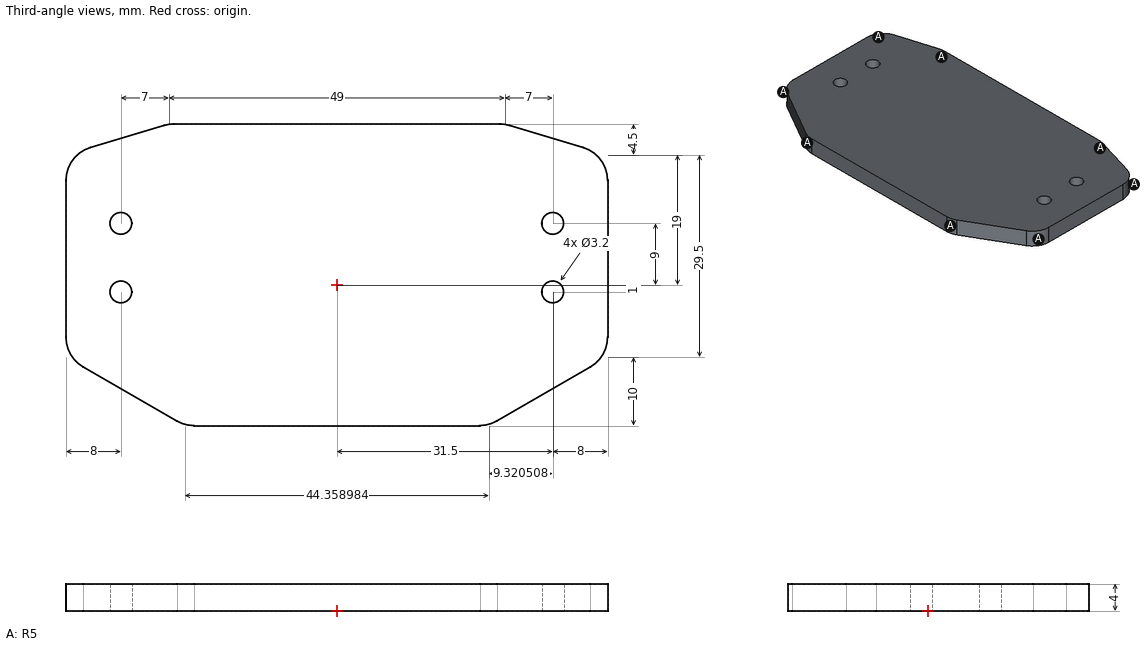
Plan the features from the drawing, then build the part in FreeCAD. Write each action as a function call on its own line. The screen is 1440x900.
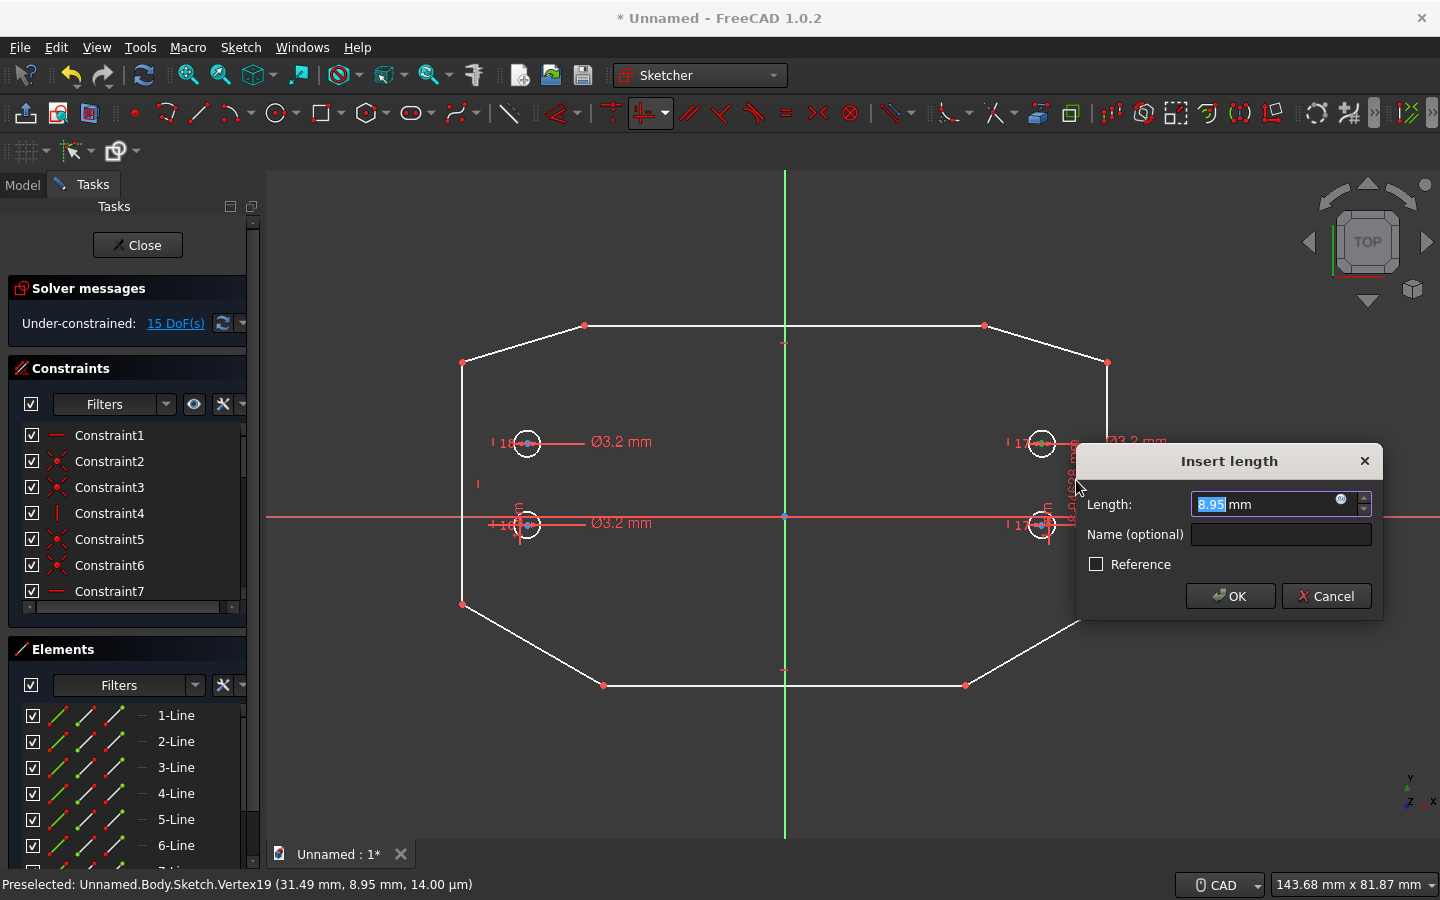
text(9)
key(Return)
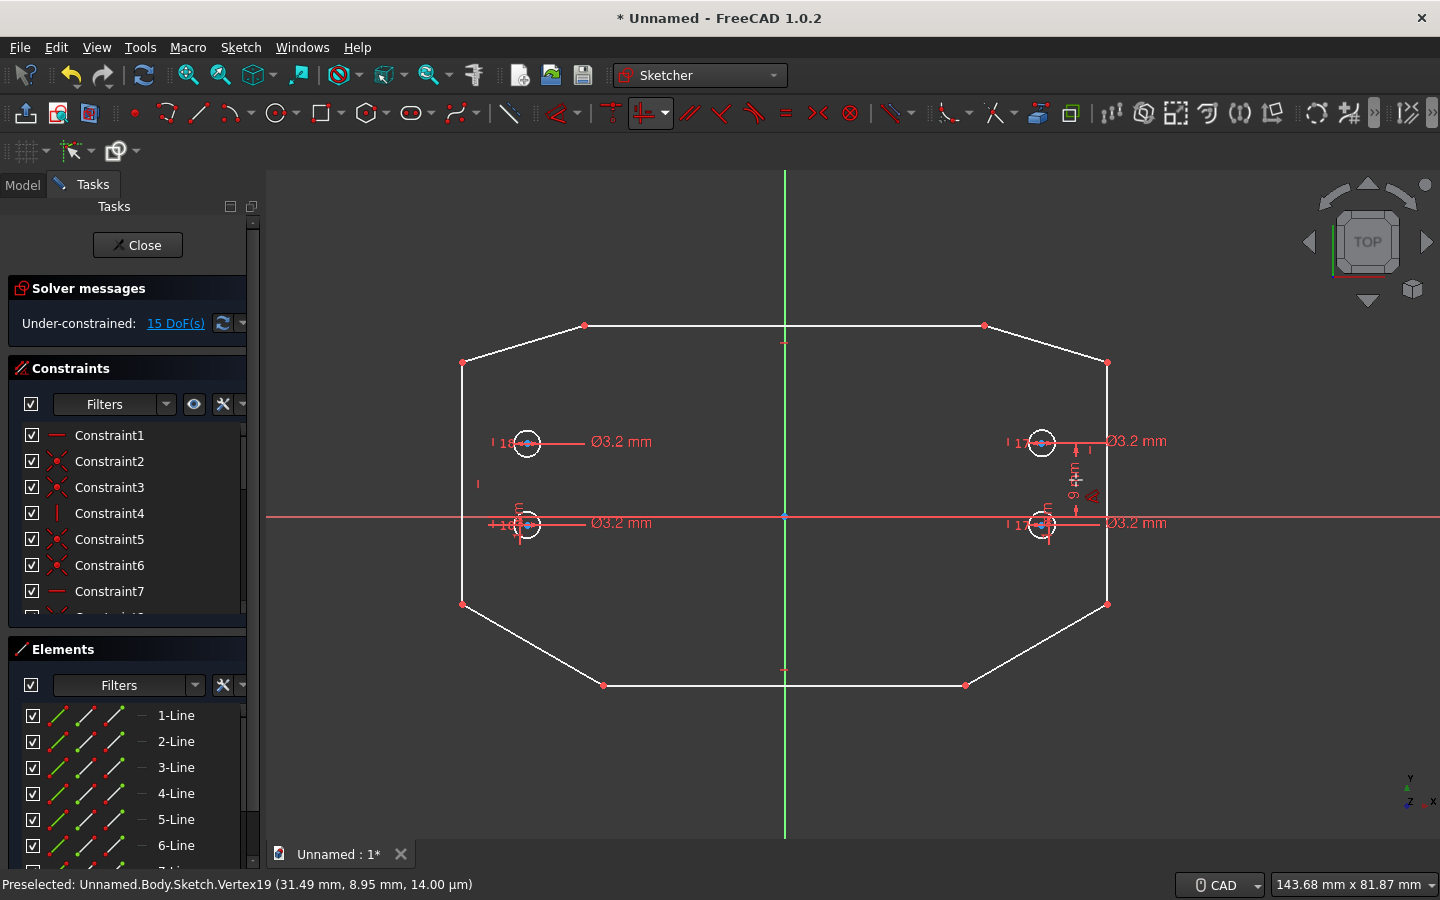
click(527, 444)
click(493, 480)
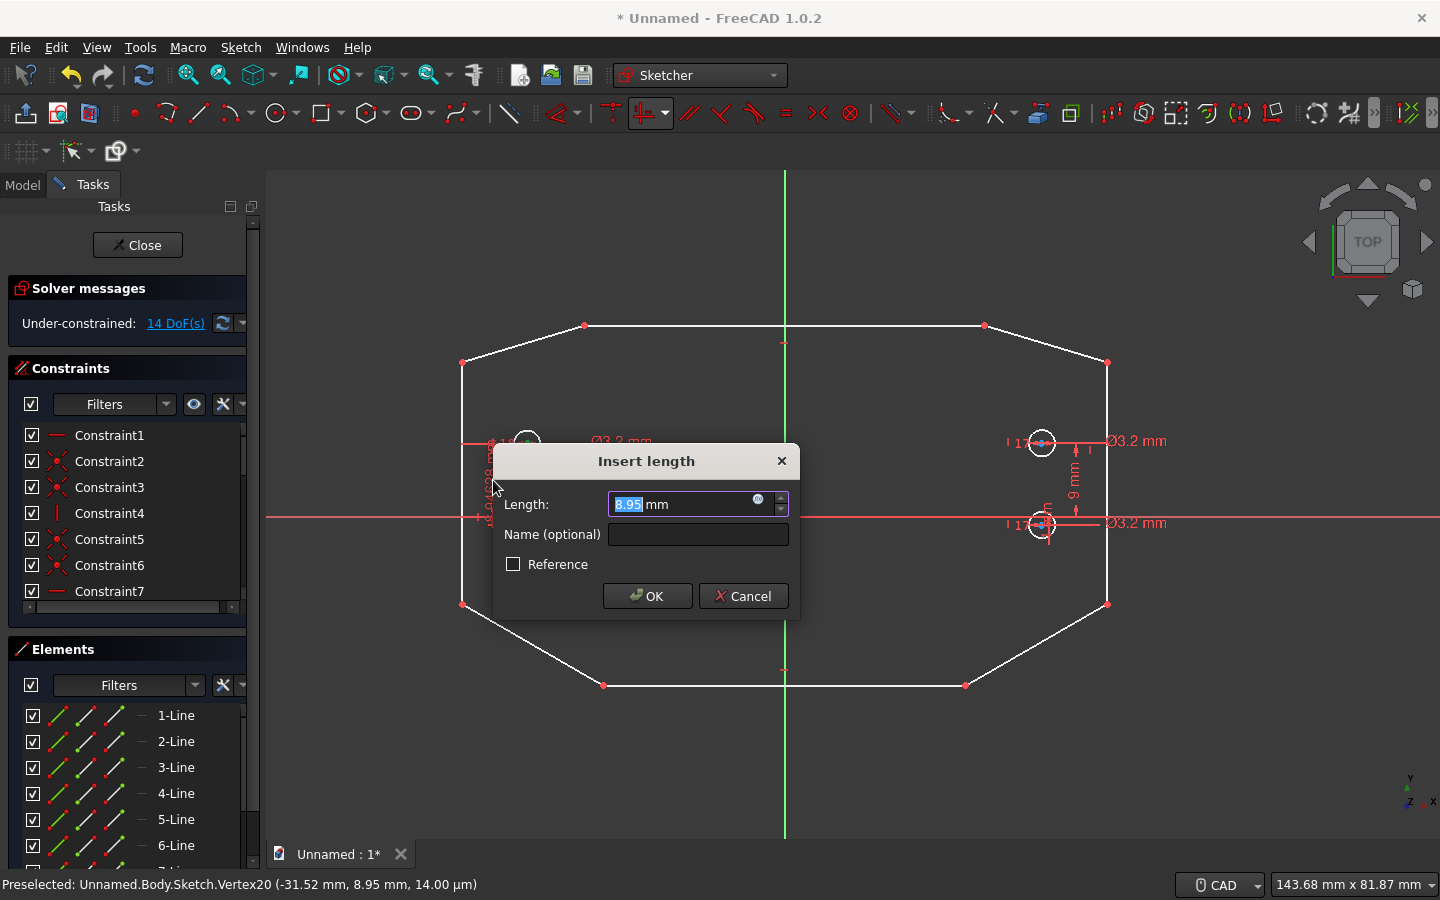
text(9)
key(Return)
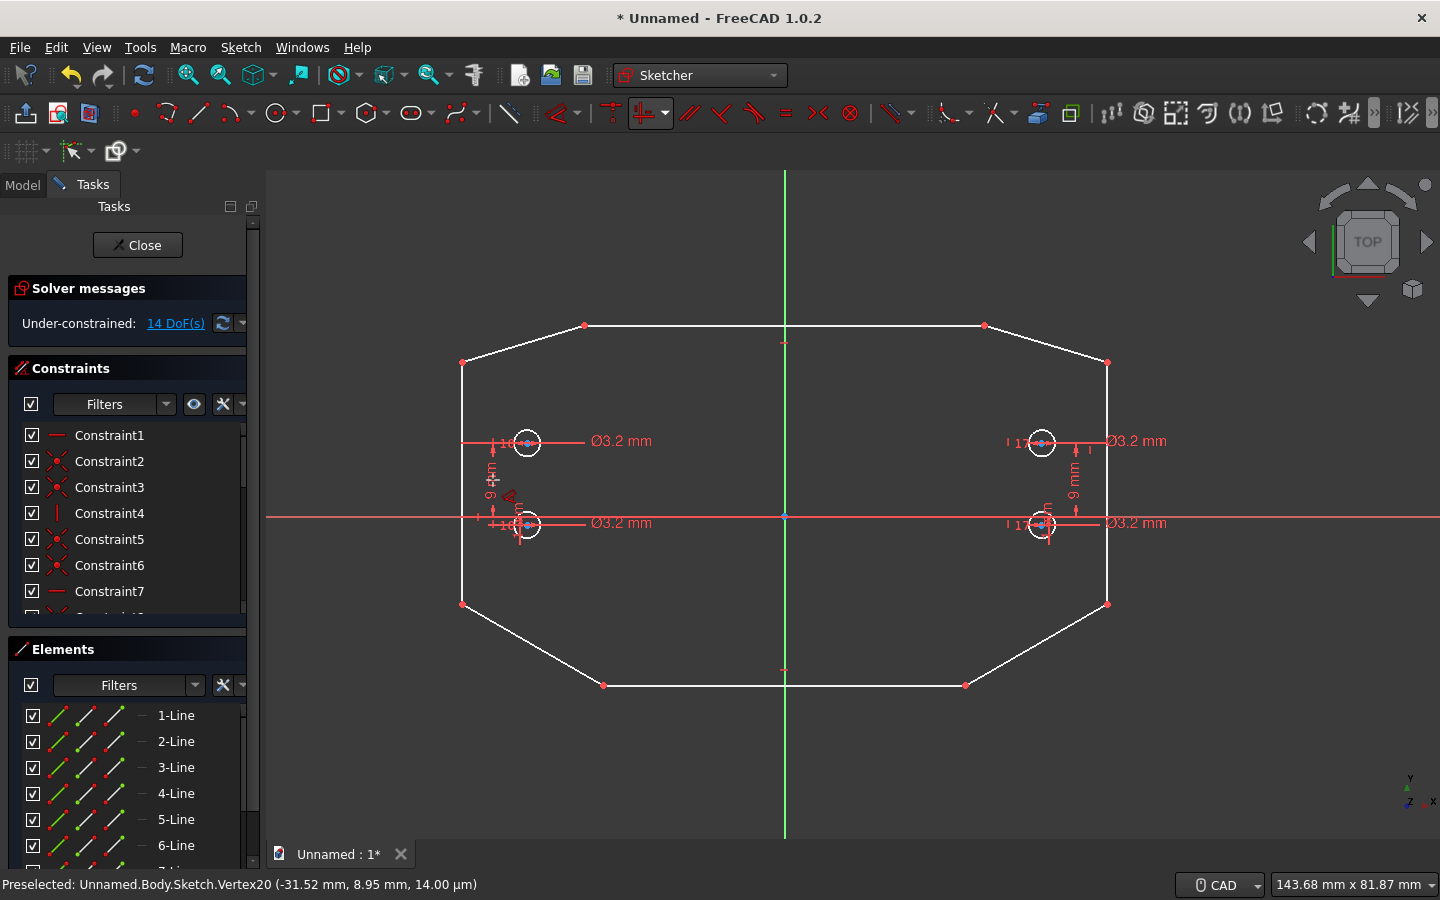
click(865, 326)
click(692, 292)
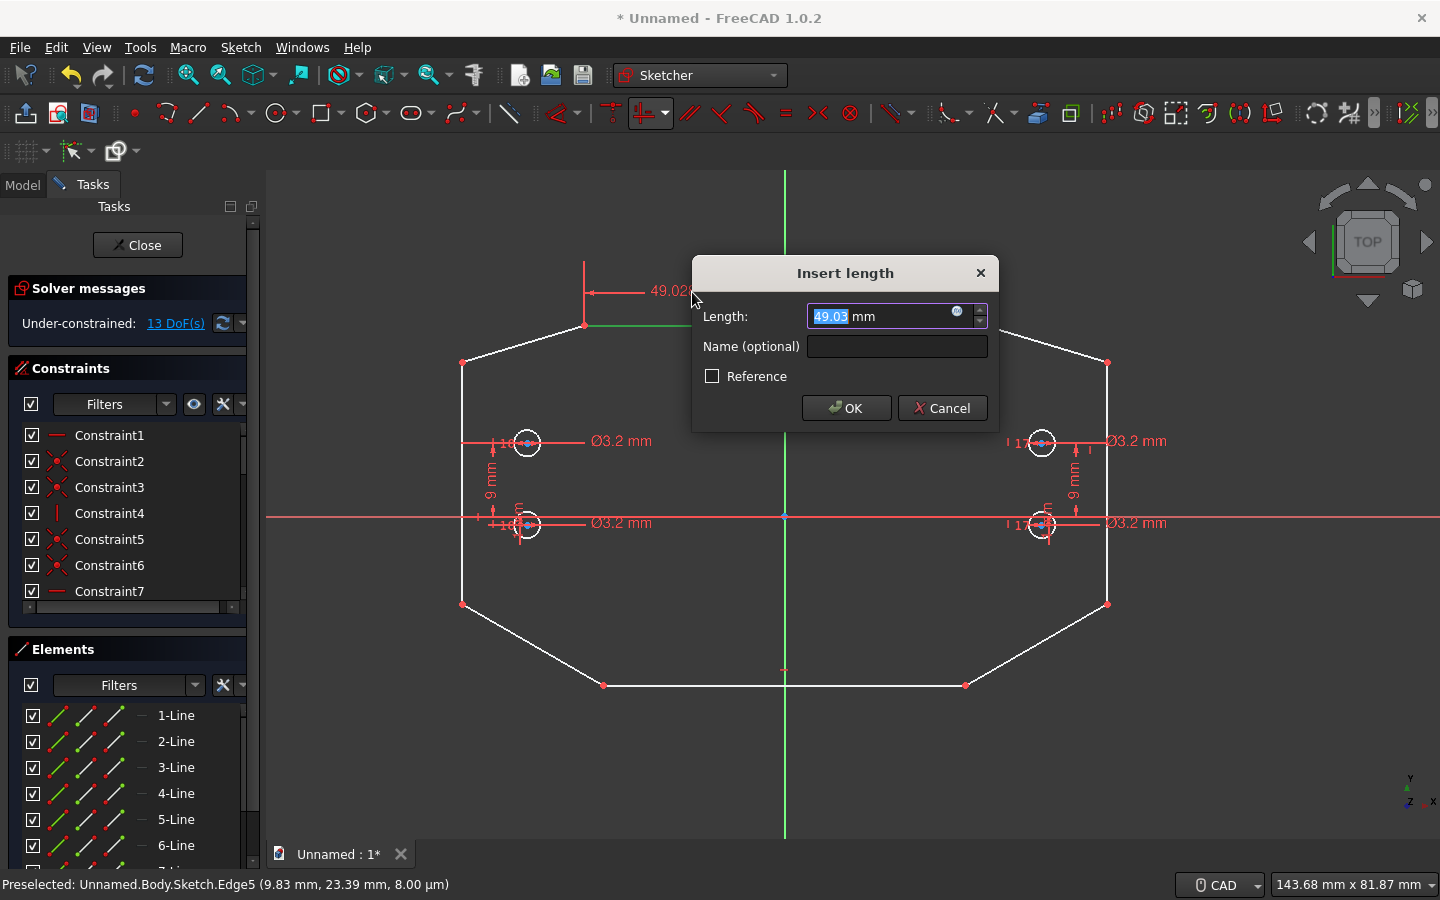
text(49)
key(Return)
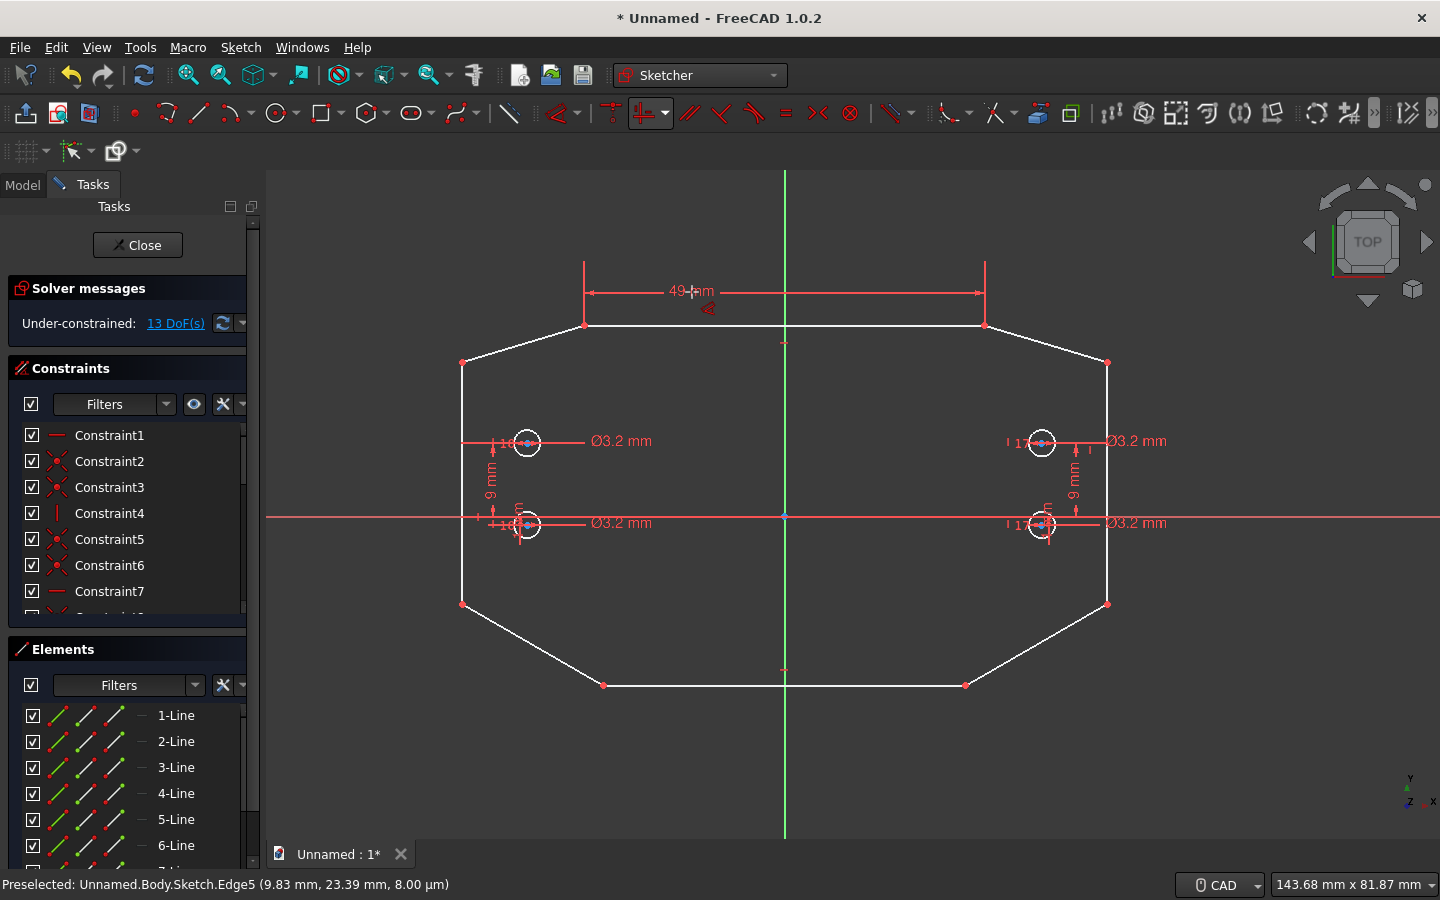
click(1107, 604)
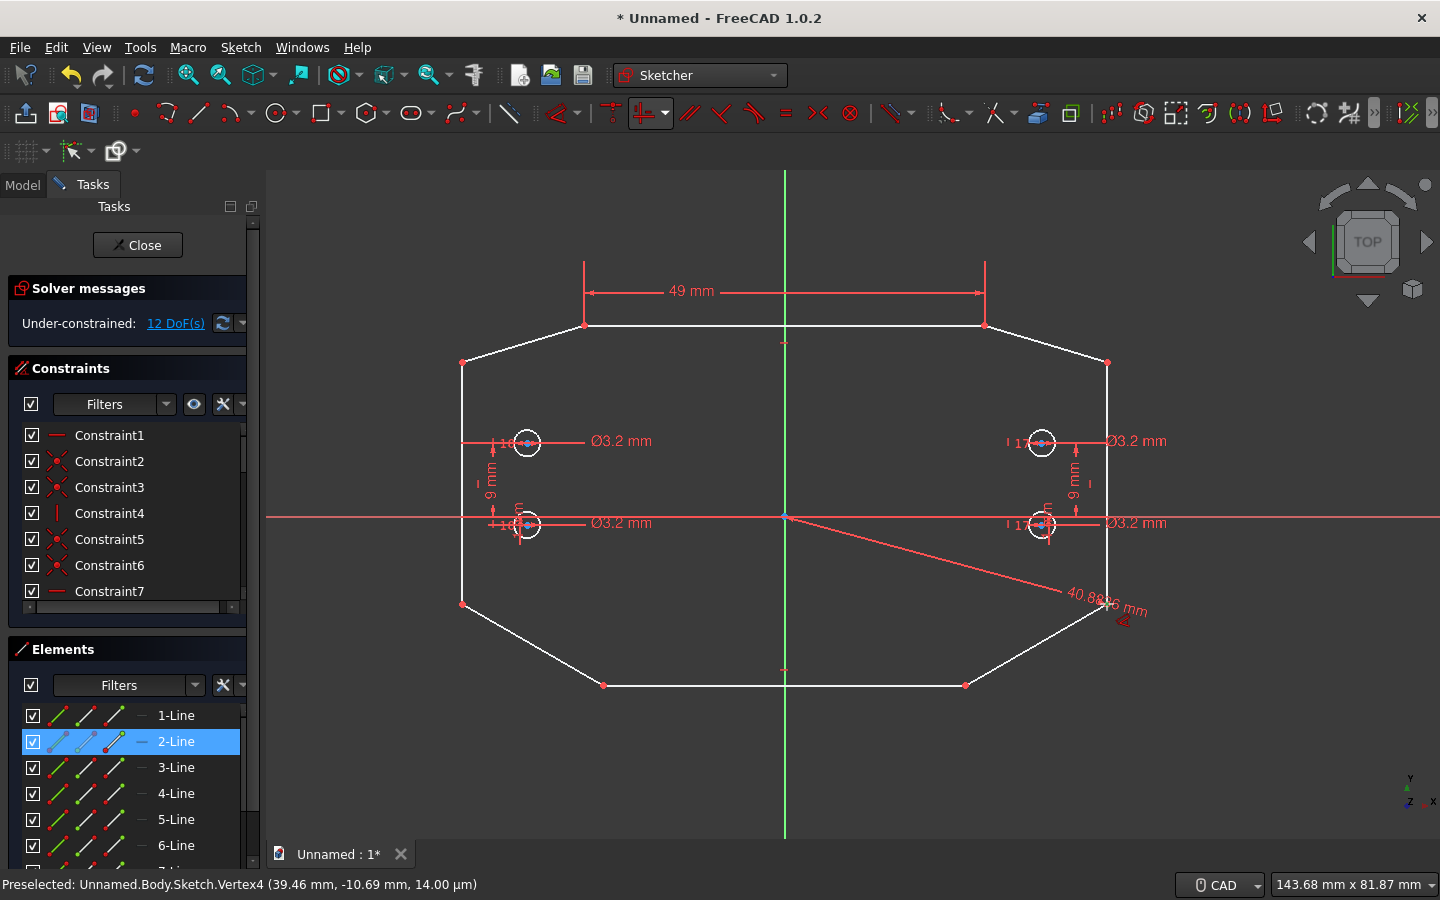
click(1042, 525)
click(1075, 638)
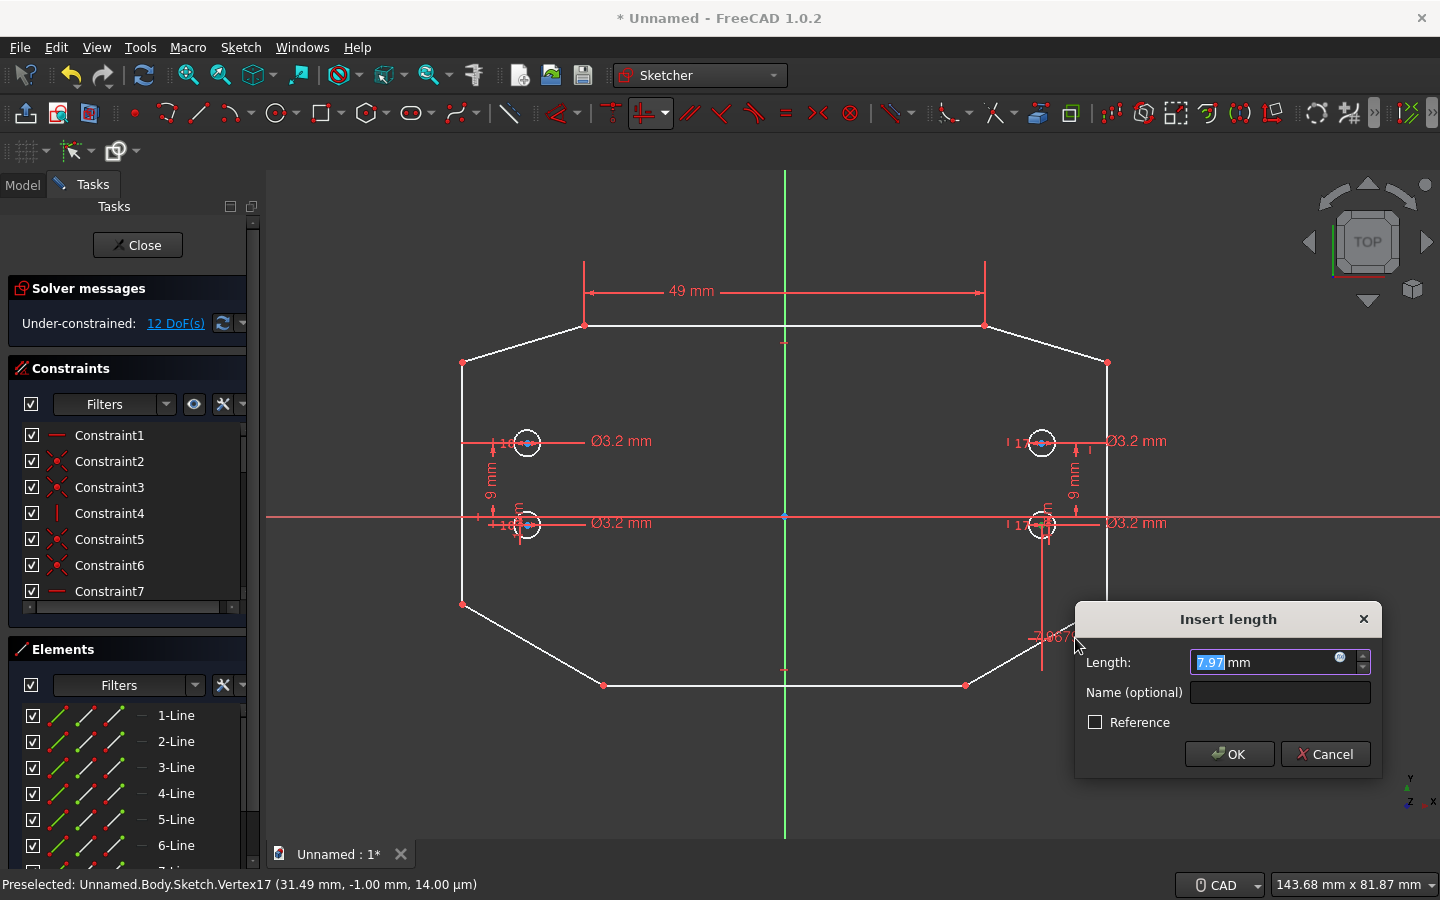
text(8)
key(Return)